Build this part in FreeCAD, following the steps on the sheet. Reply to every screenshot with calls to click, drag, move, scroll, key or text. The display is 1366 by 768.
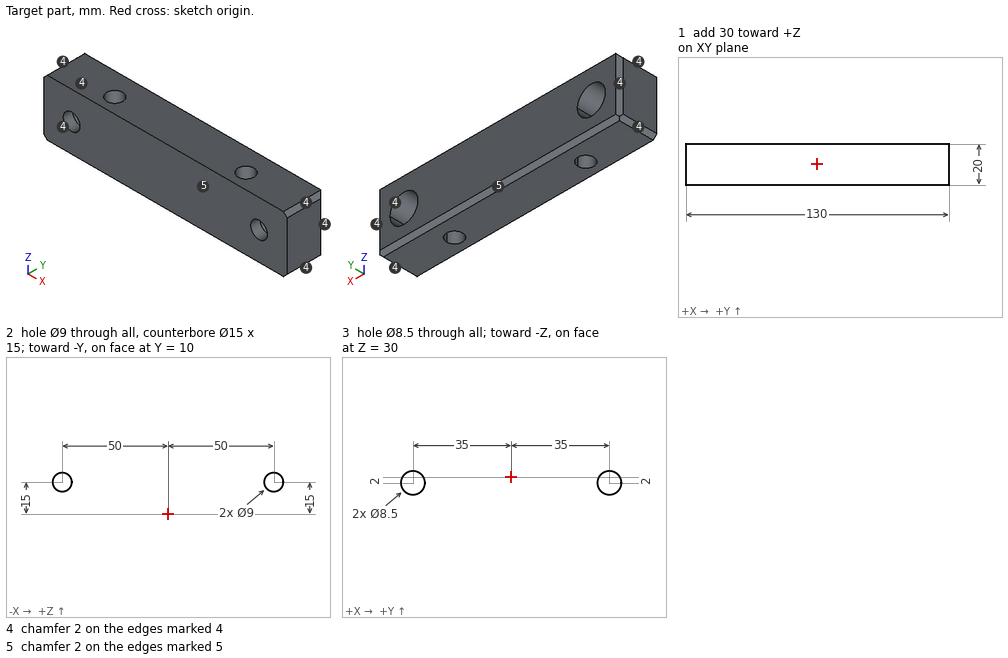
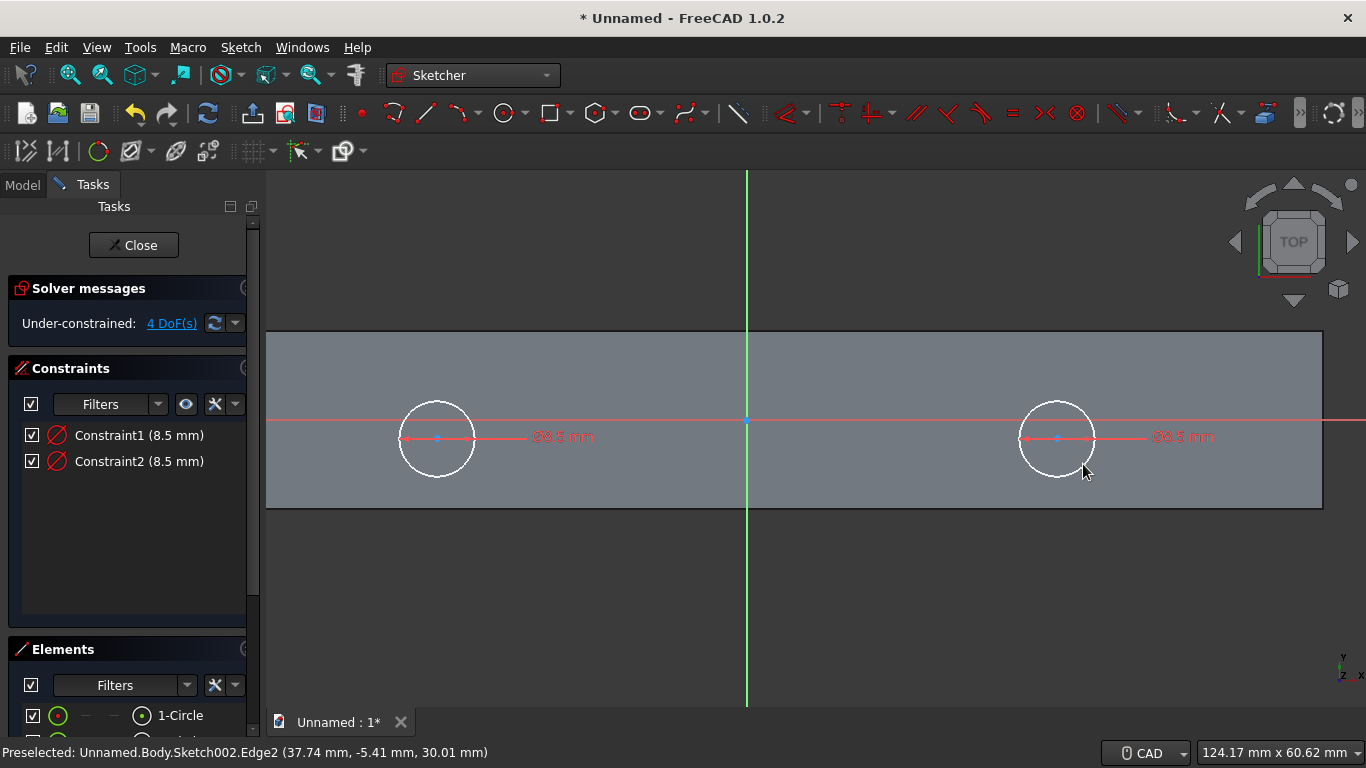
click(786, 114)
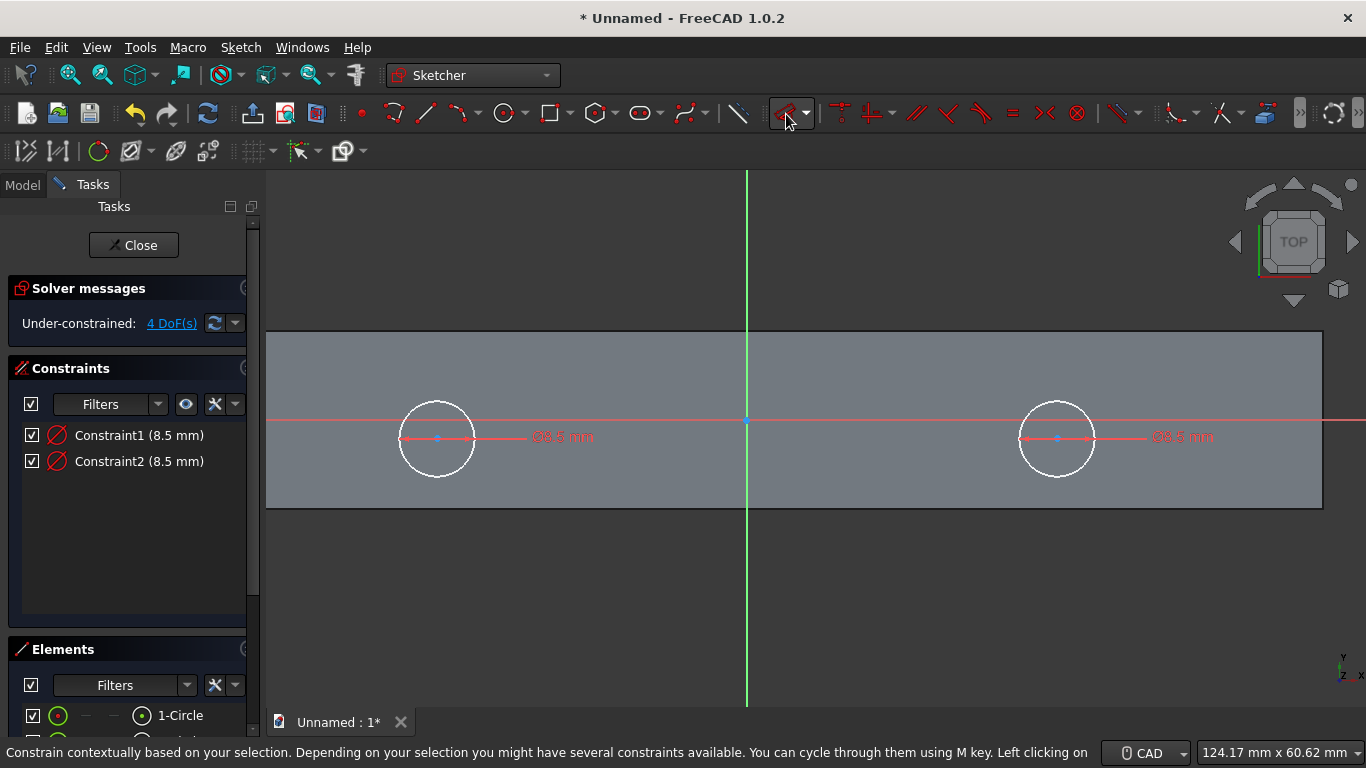
scroll(437, 439, up, 5)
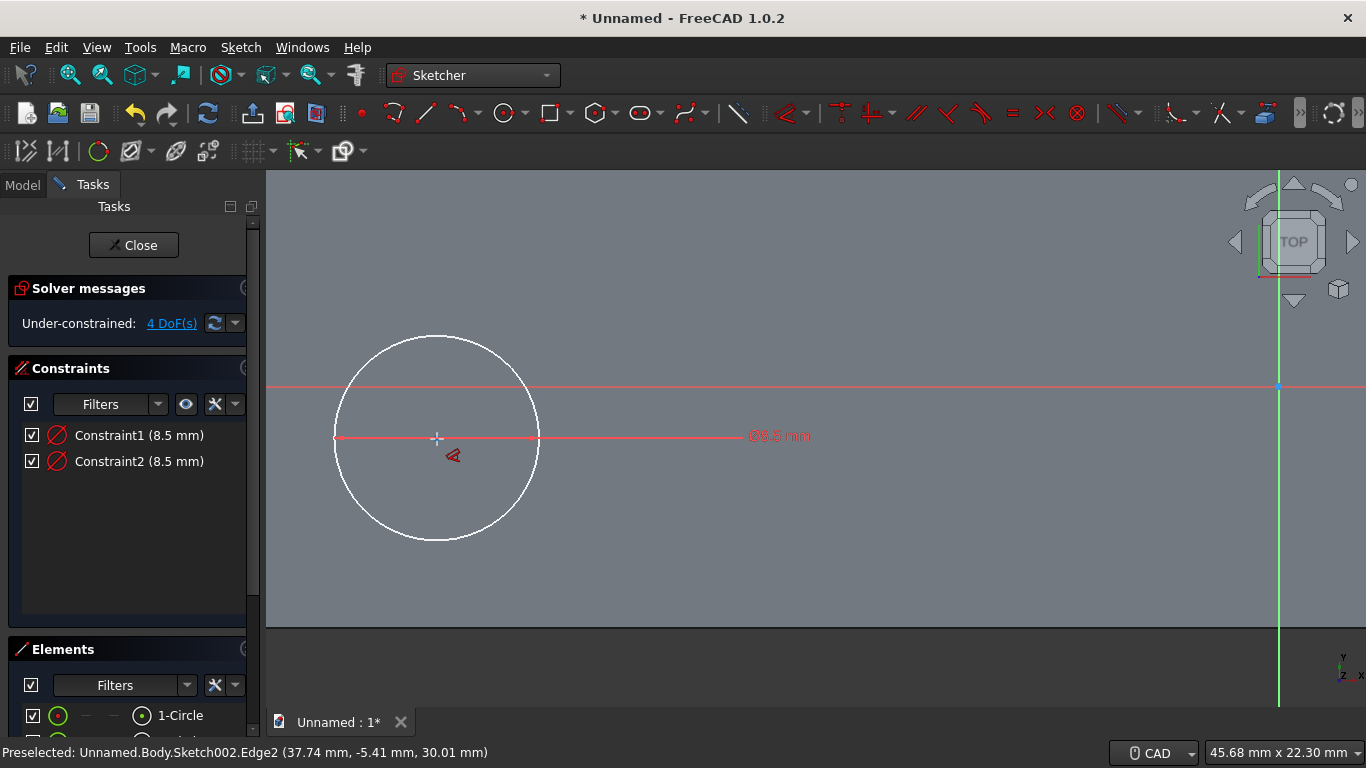
click(437, 438)
click(403, 412)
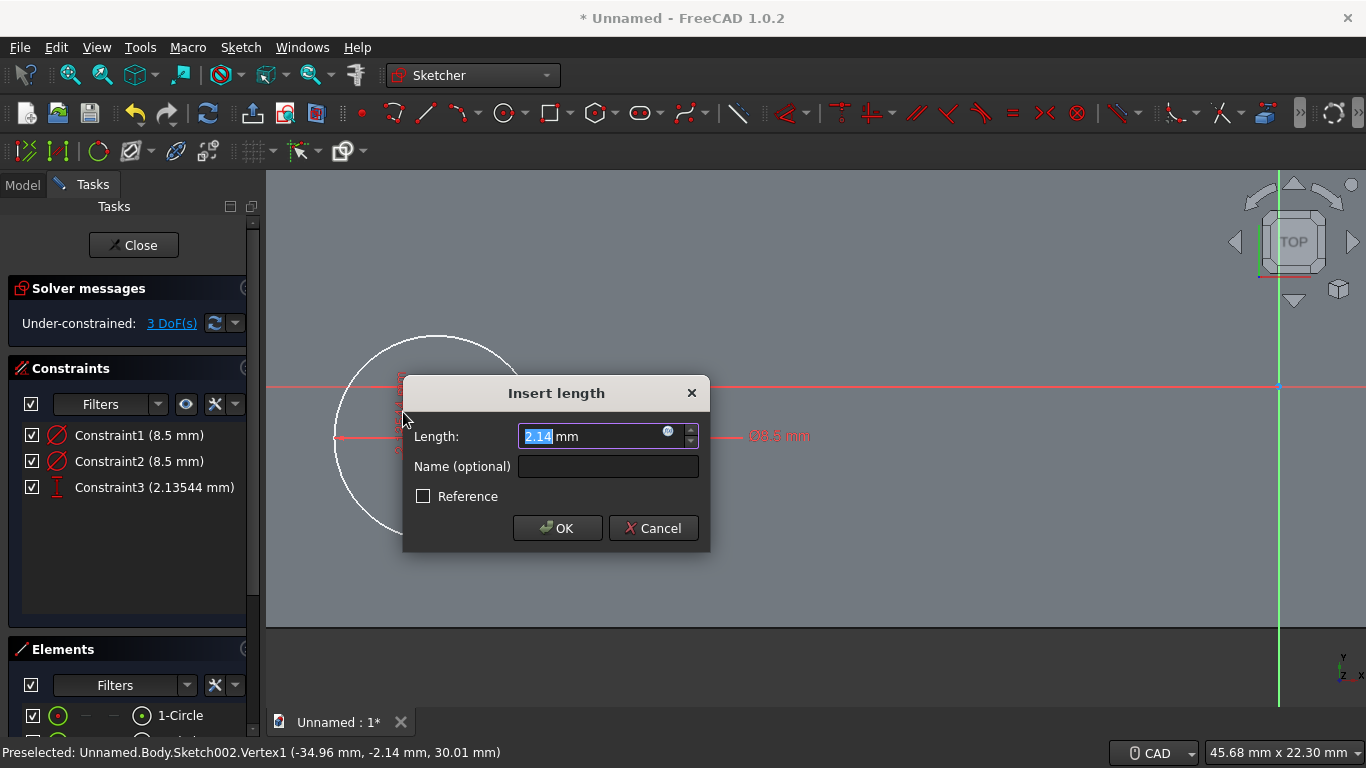
text(2)
key(Return)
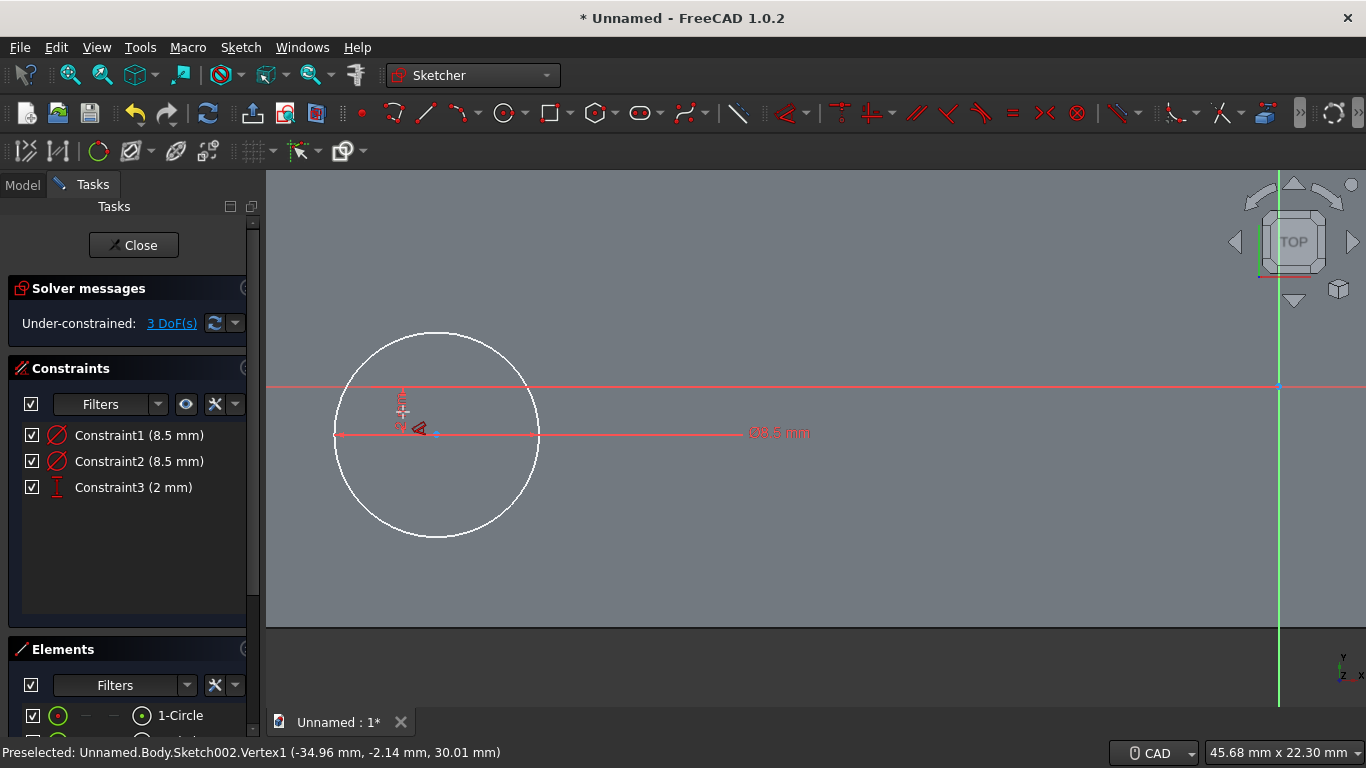
scroll(438, 441, down, 5)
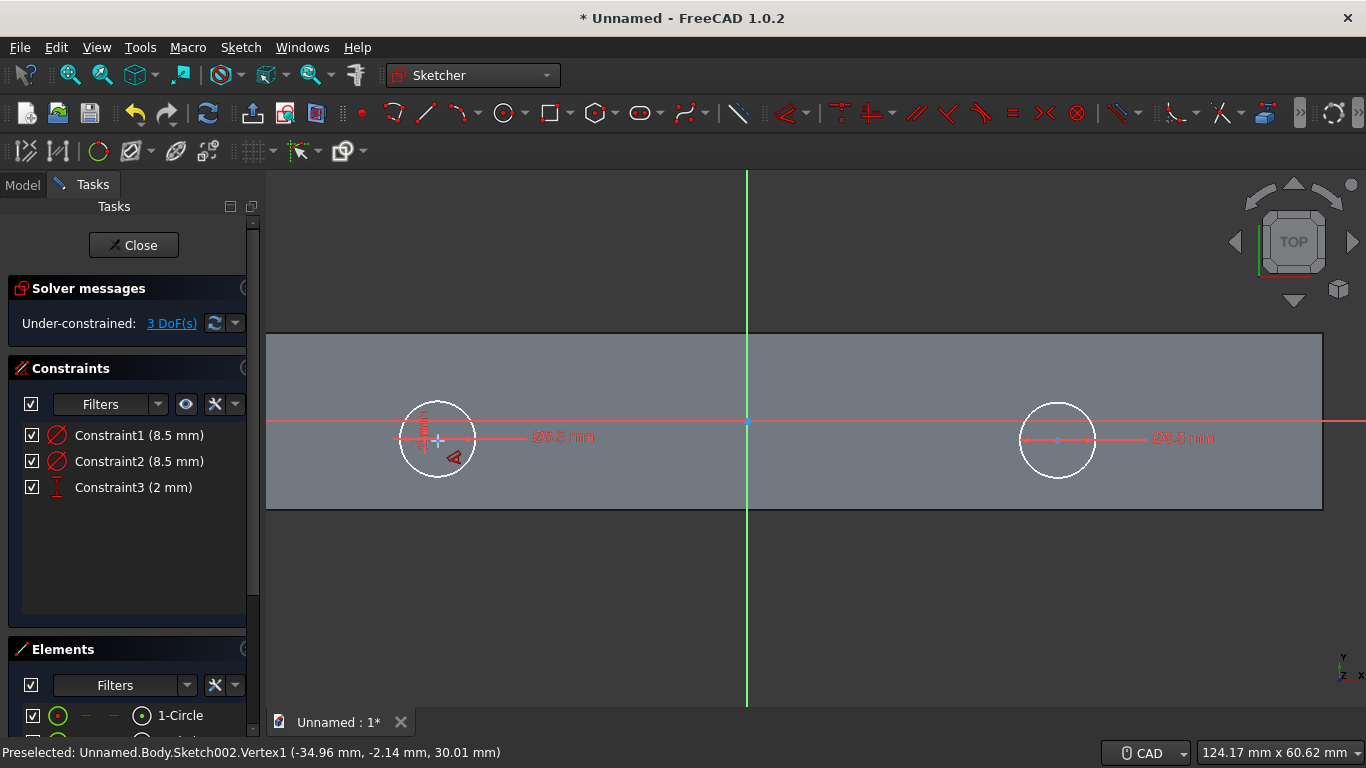
scroll(1058, 440, up, 5)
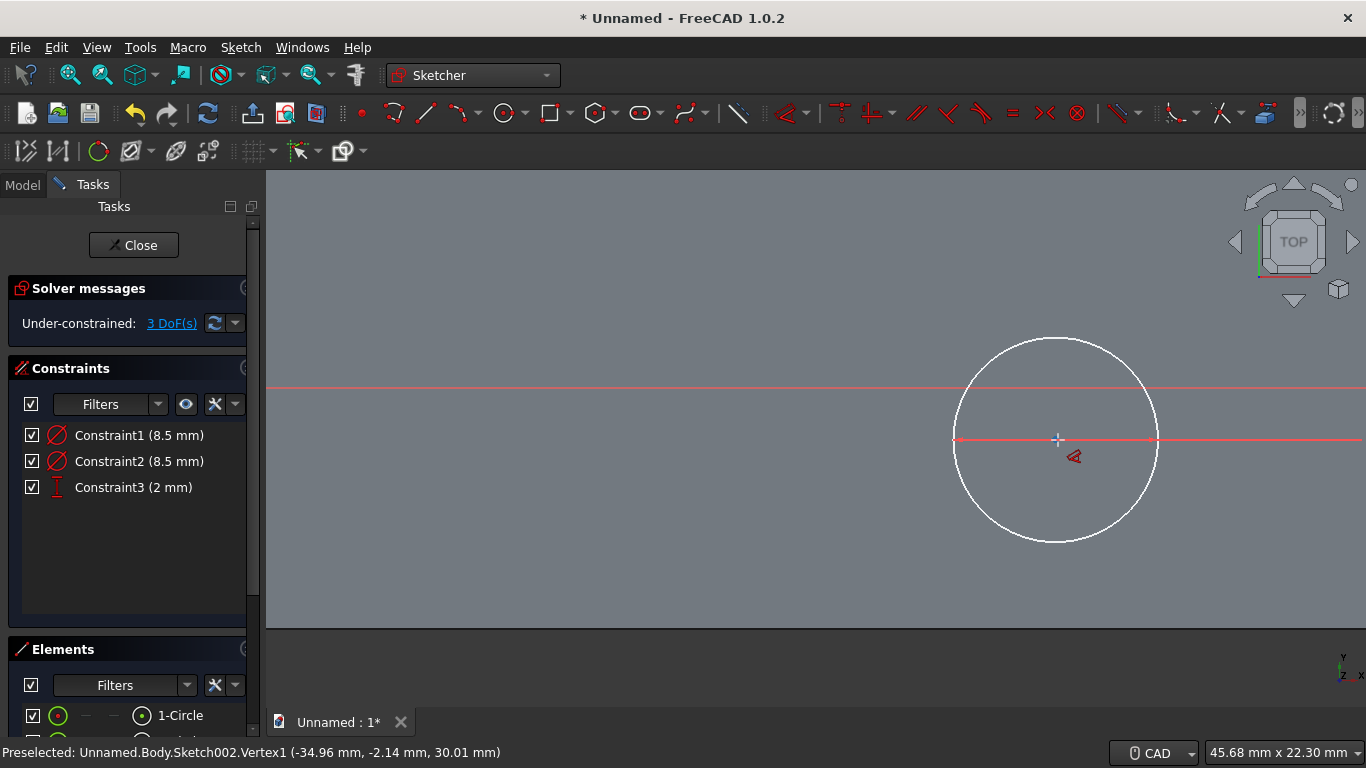
click(1056, 440)
click(1090, 414)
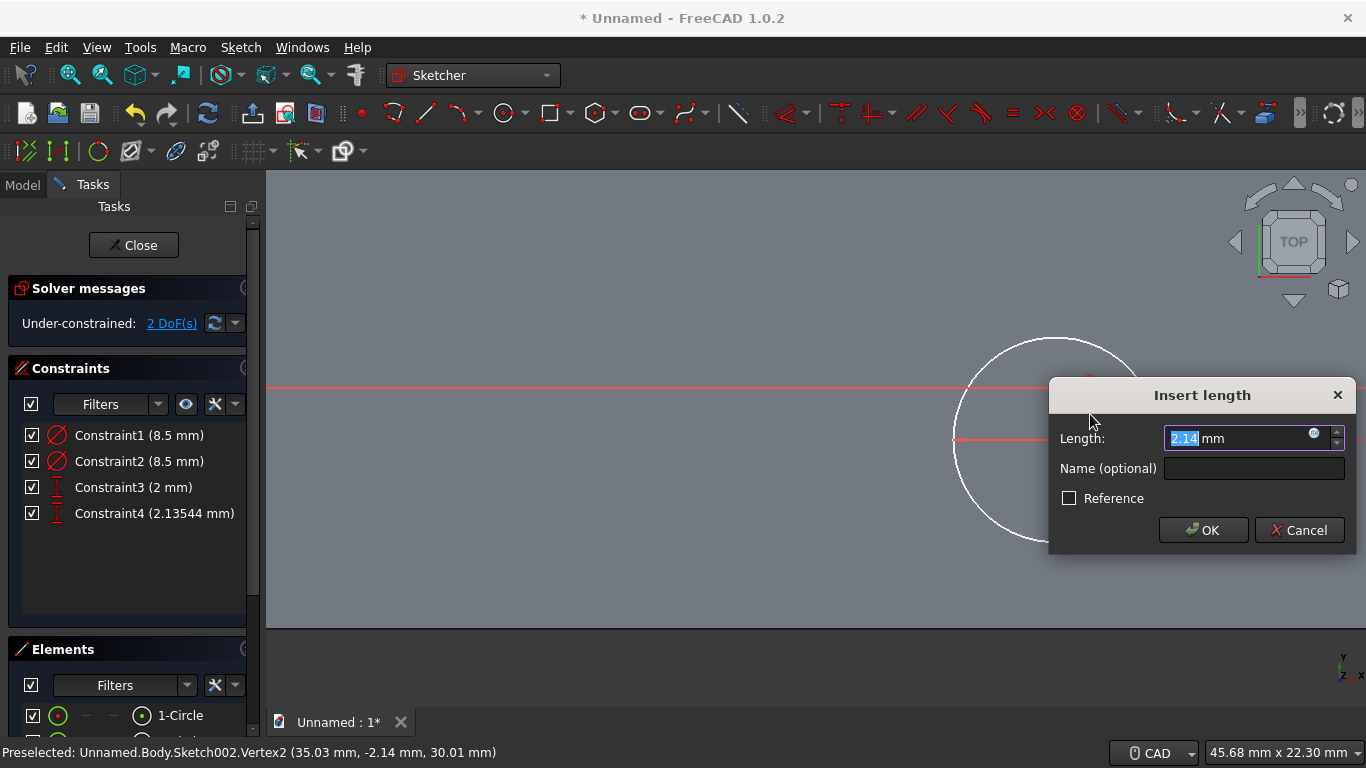
text(2)
key(Return)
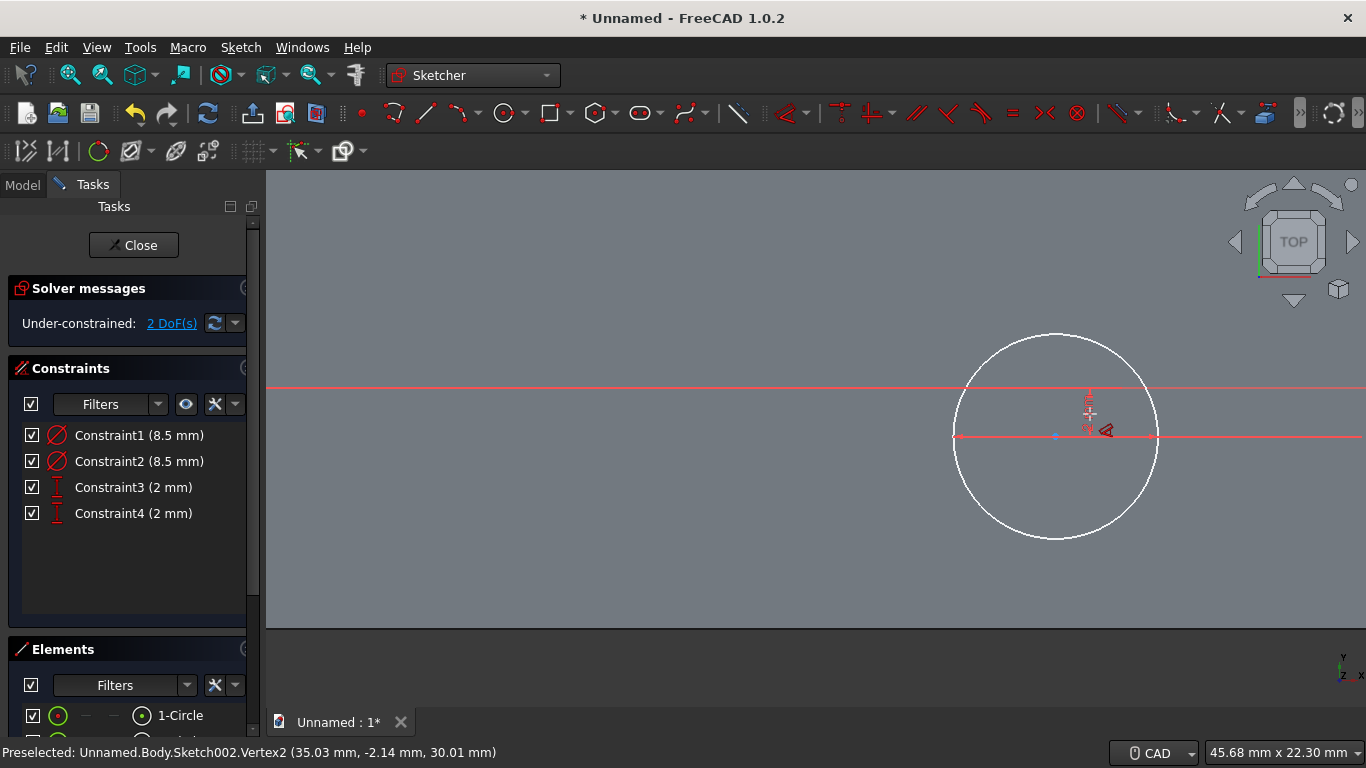
scroll(1059, 440, down, 5)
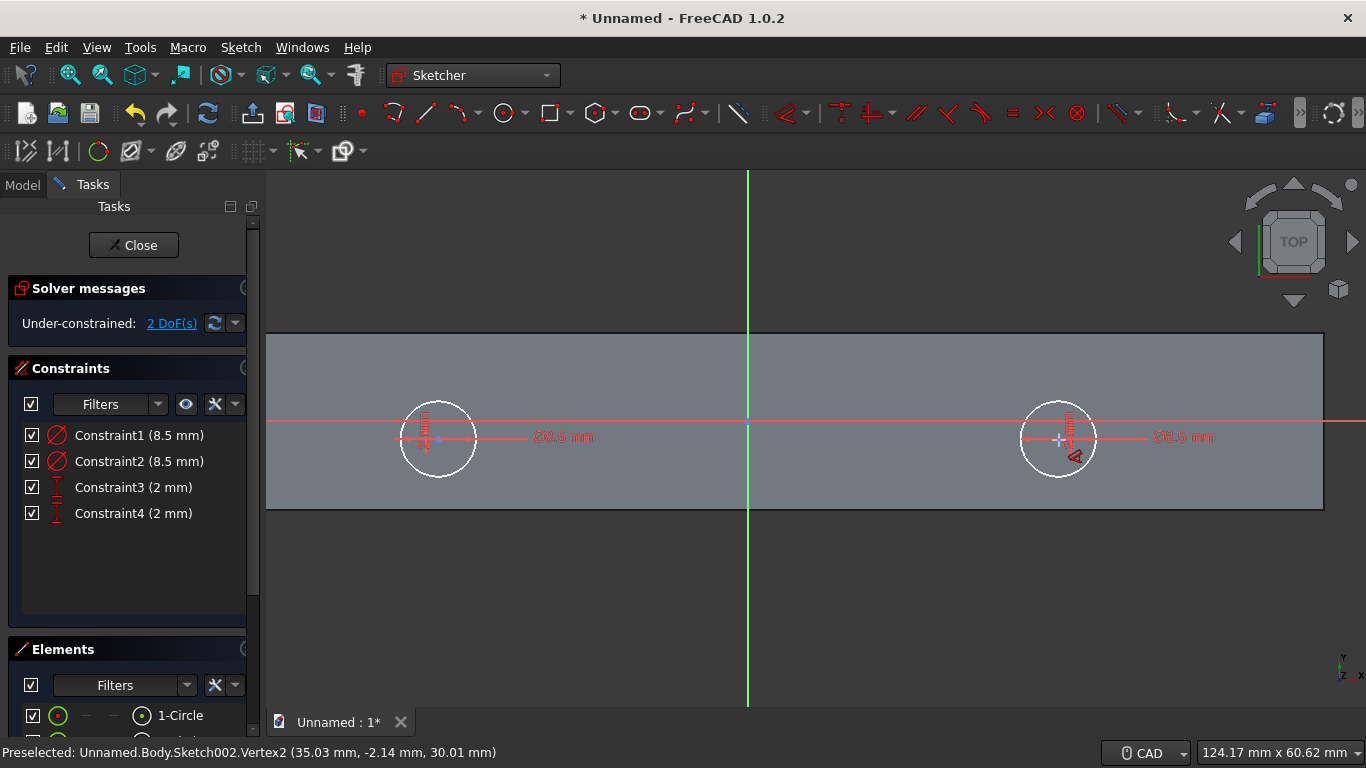
click(438, 439)
click(593, 387)